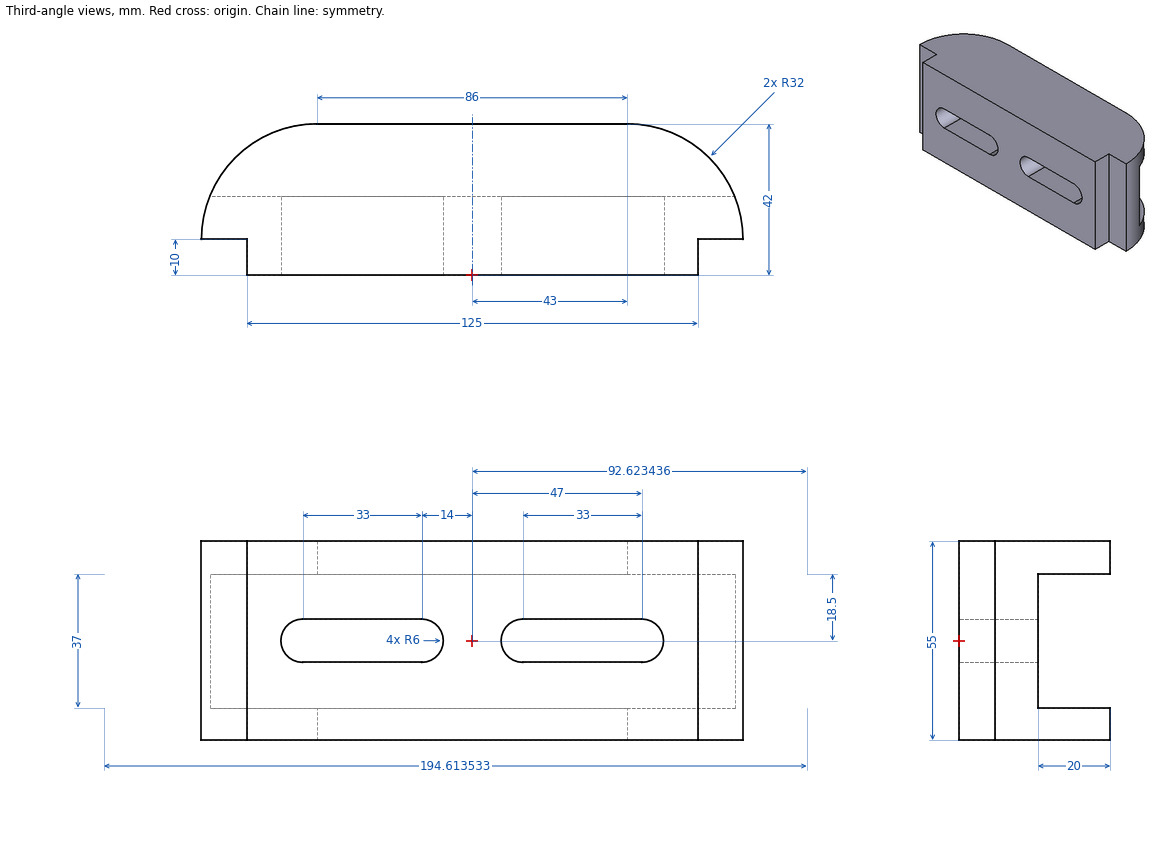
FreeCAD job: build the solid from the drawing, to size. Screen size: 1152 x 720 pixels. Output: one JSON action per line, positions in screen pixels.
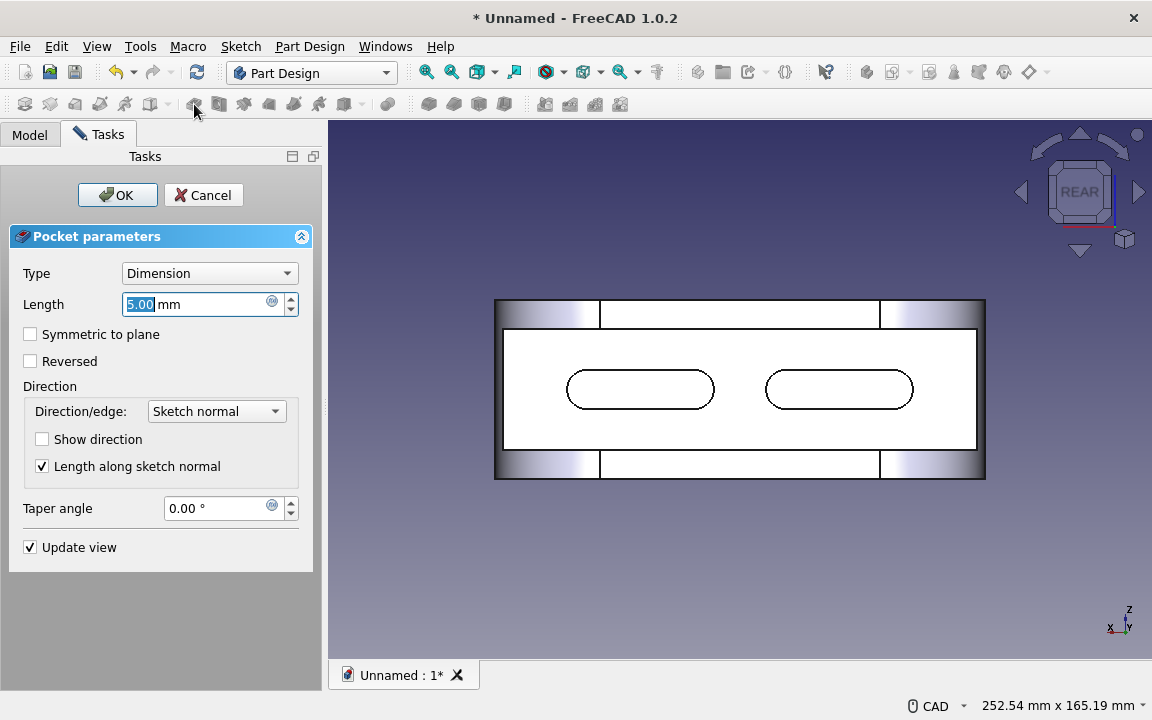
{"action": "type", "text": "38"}
{"action": "key", "text": "Tab"}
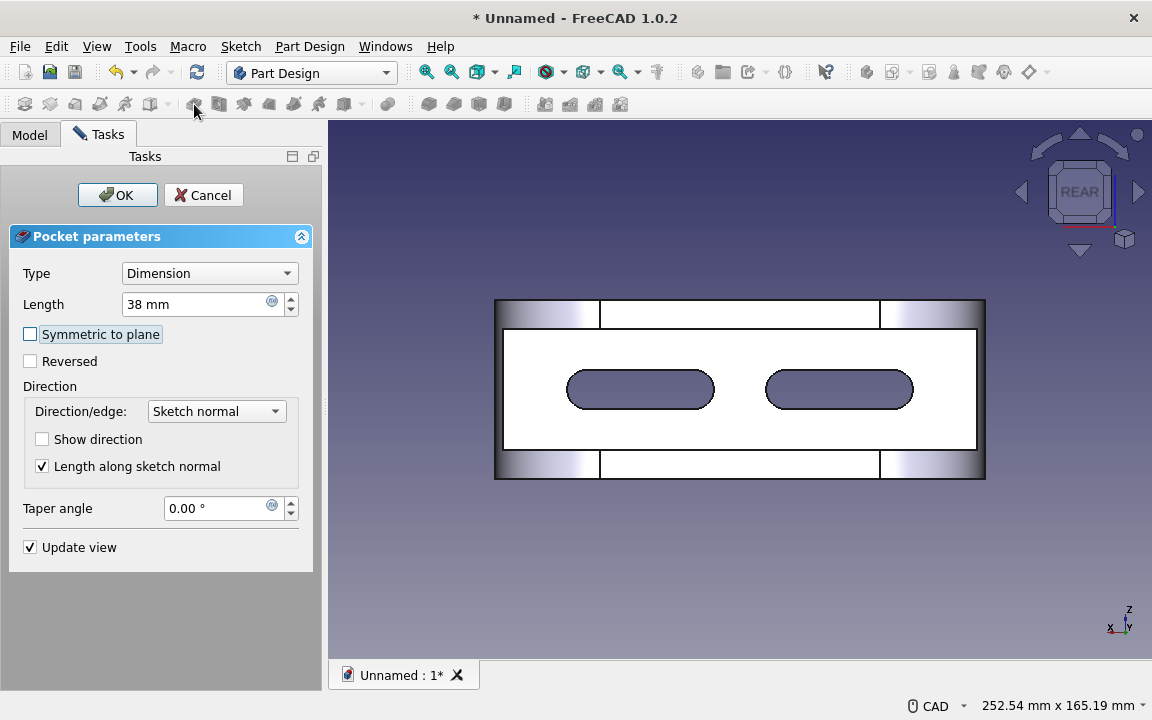
{"action": "left_click", "coordinate": [118, 195]}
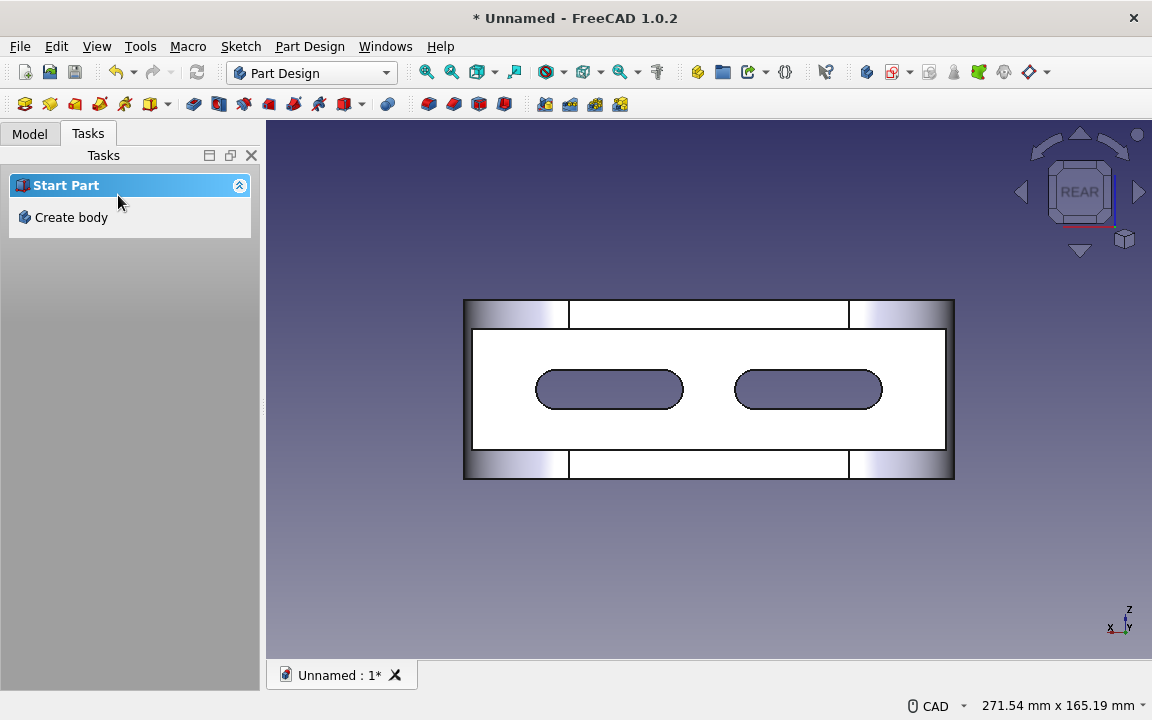
{"action": "key", "text": "0"}